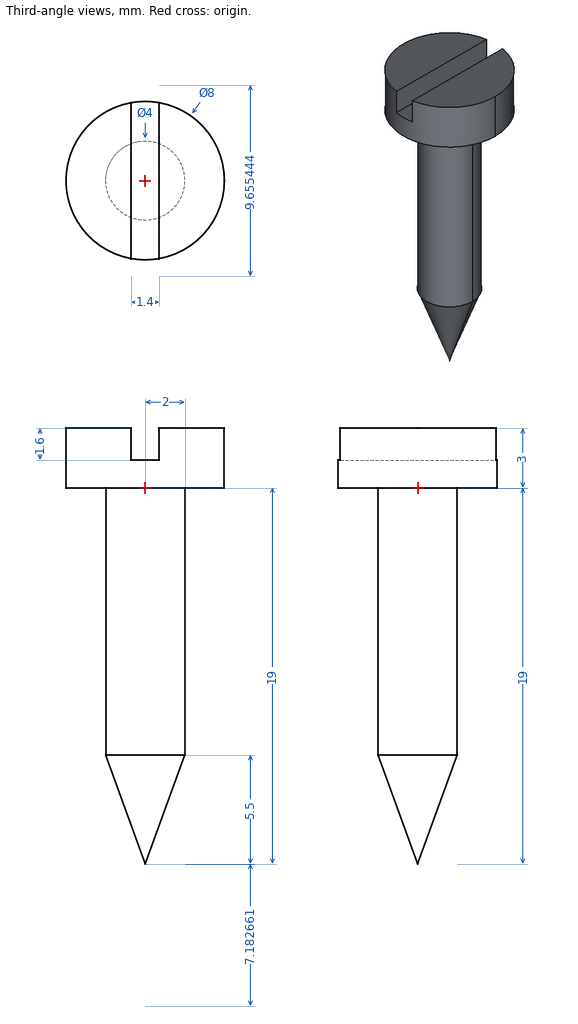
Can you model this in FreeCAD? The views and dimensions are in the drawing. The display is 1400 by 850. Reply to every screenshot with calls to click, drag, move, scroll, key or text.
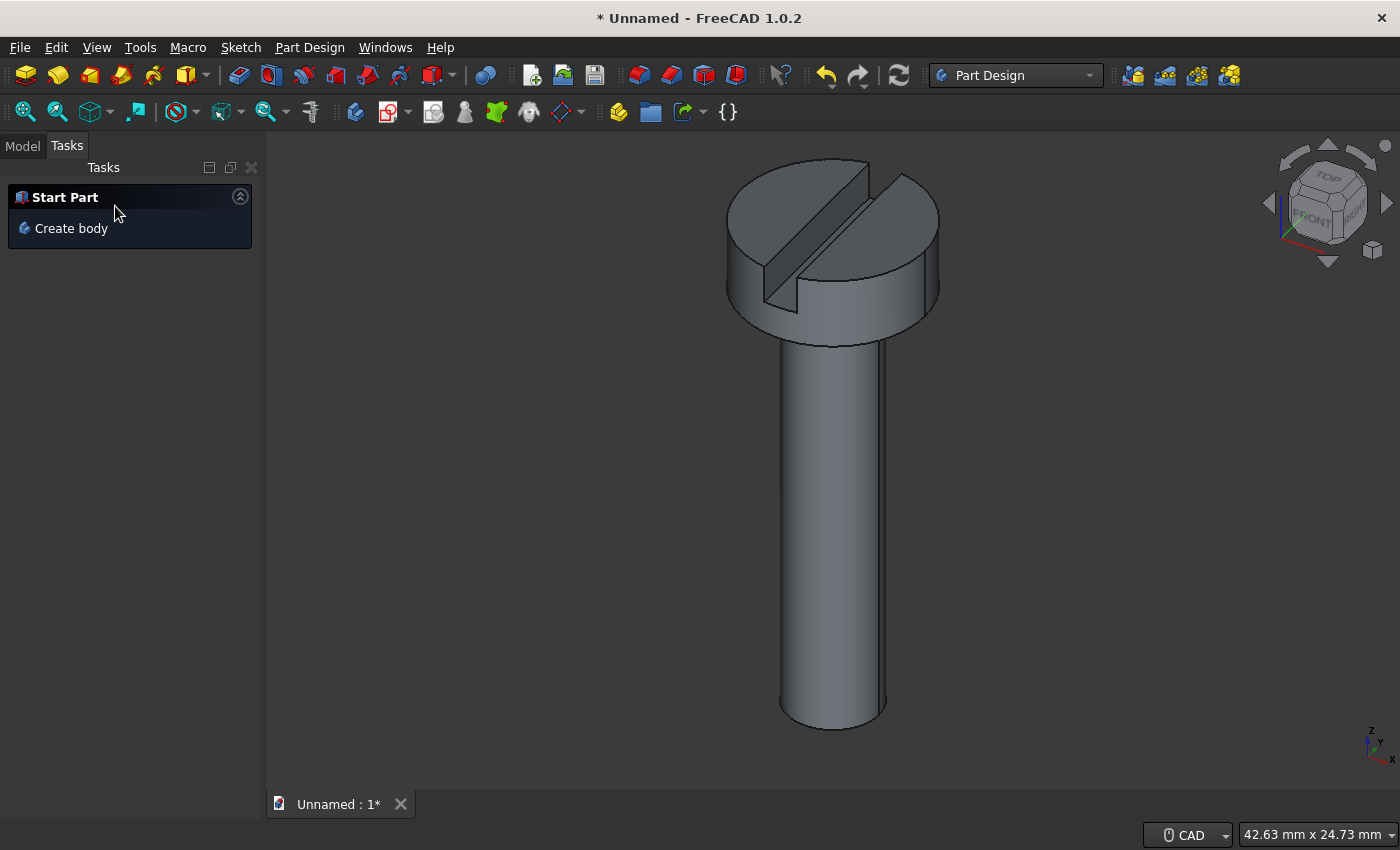
click(388, 112)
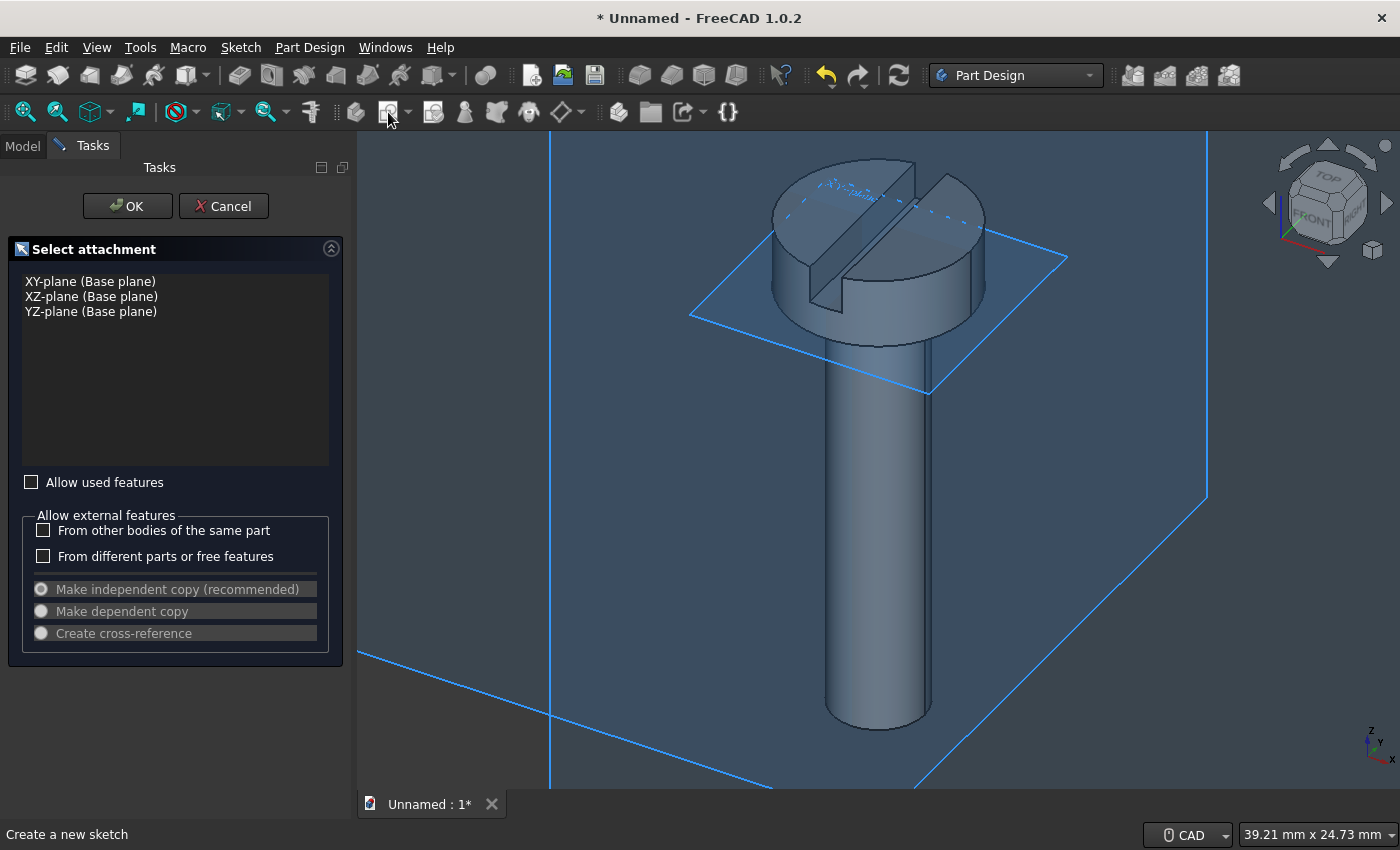
click(82, 296)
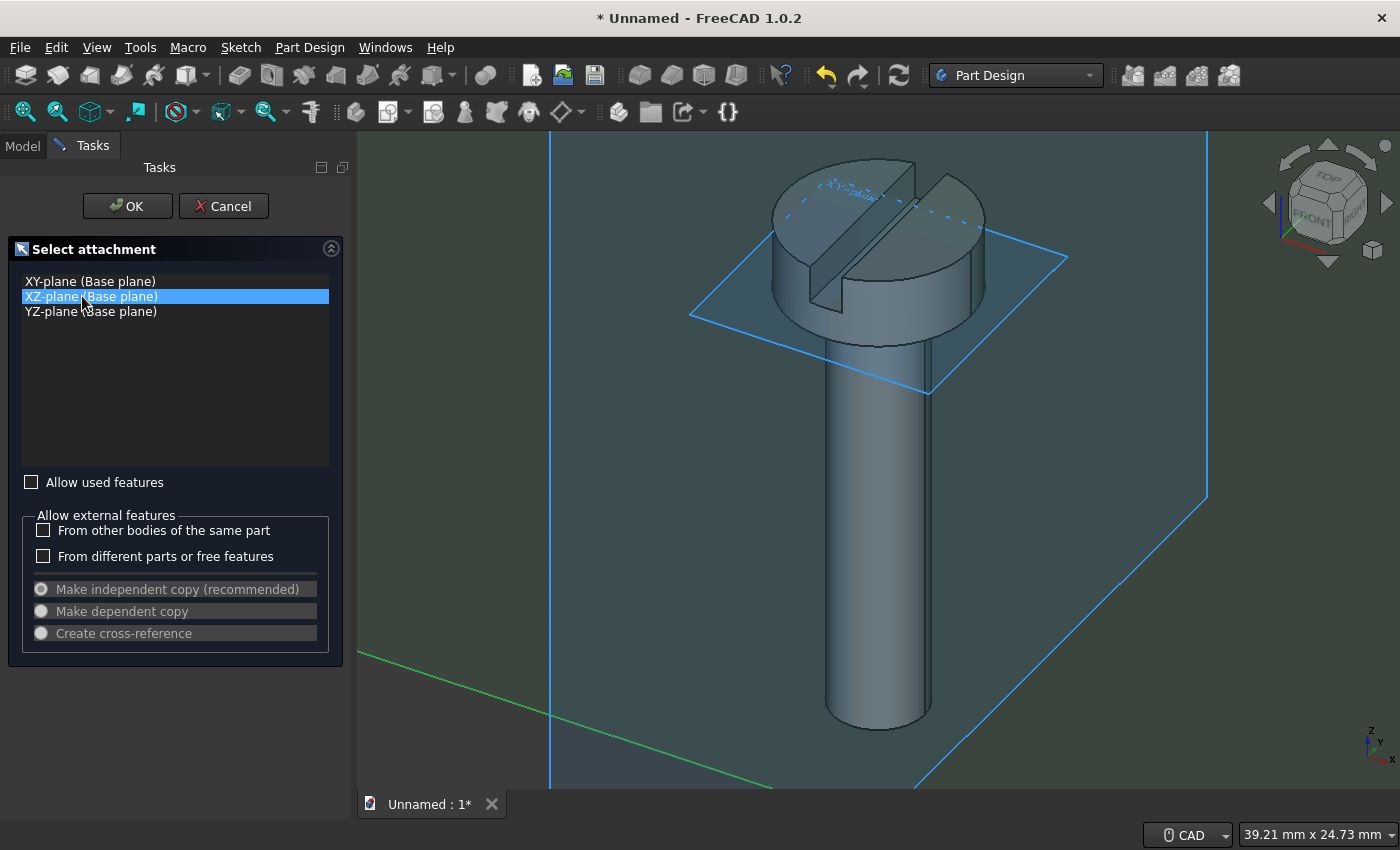
click(128, 206)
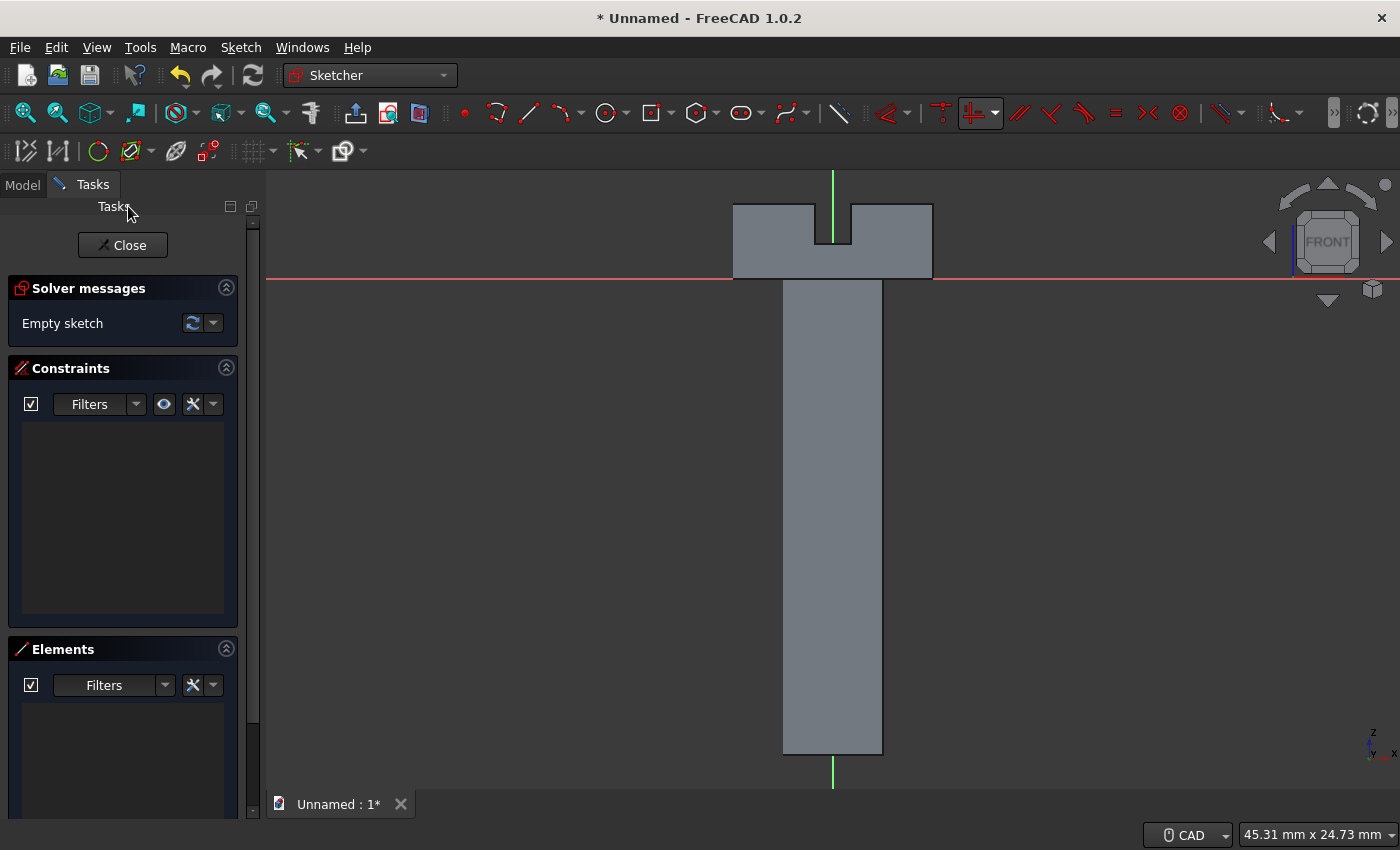
key(q)
key(s)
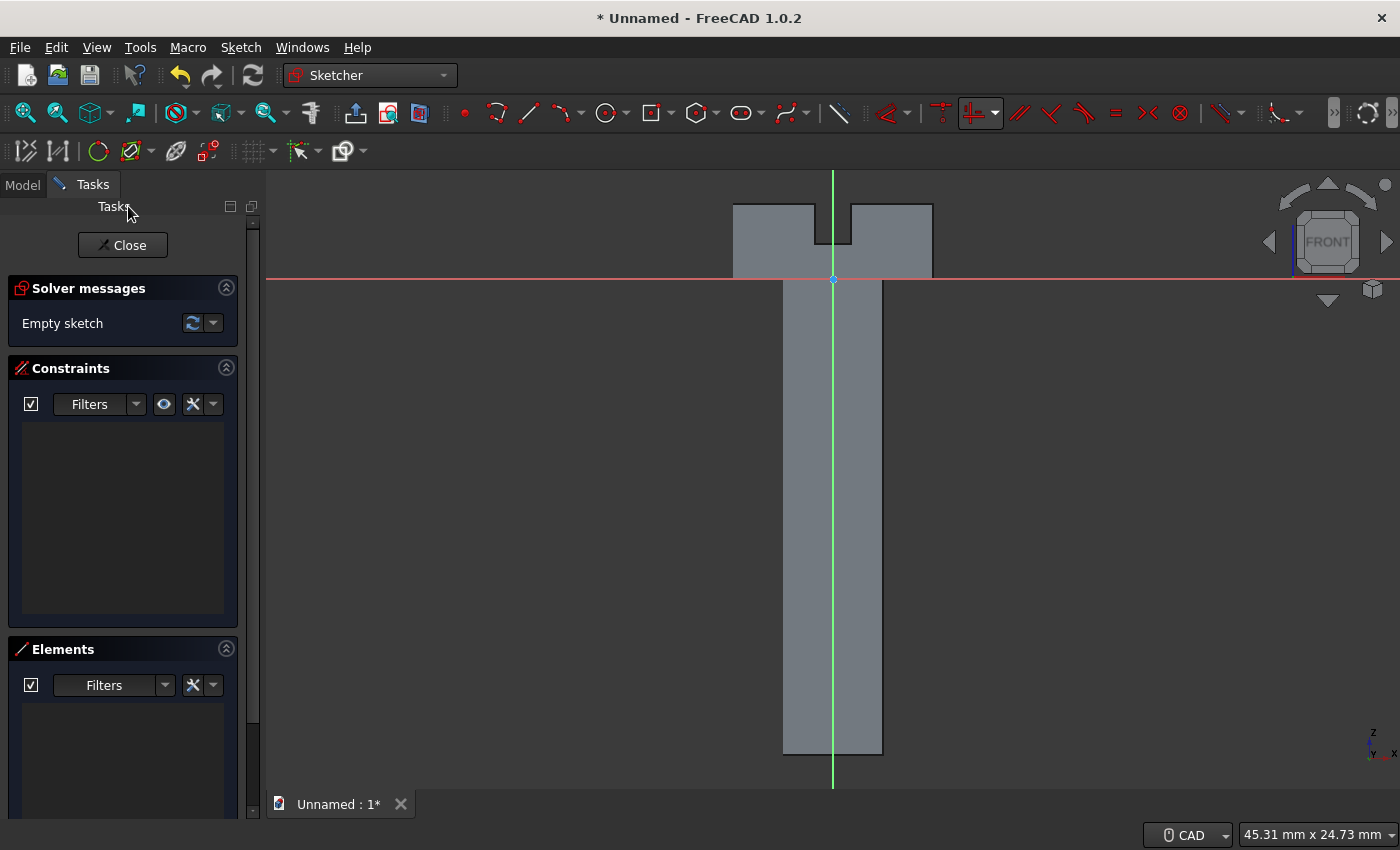
scroll(651, 325, down, 3)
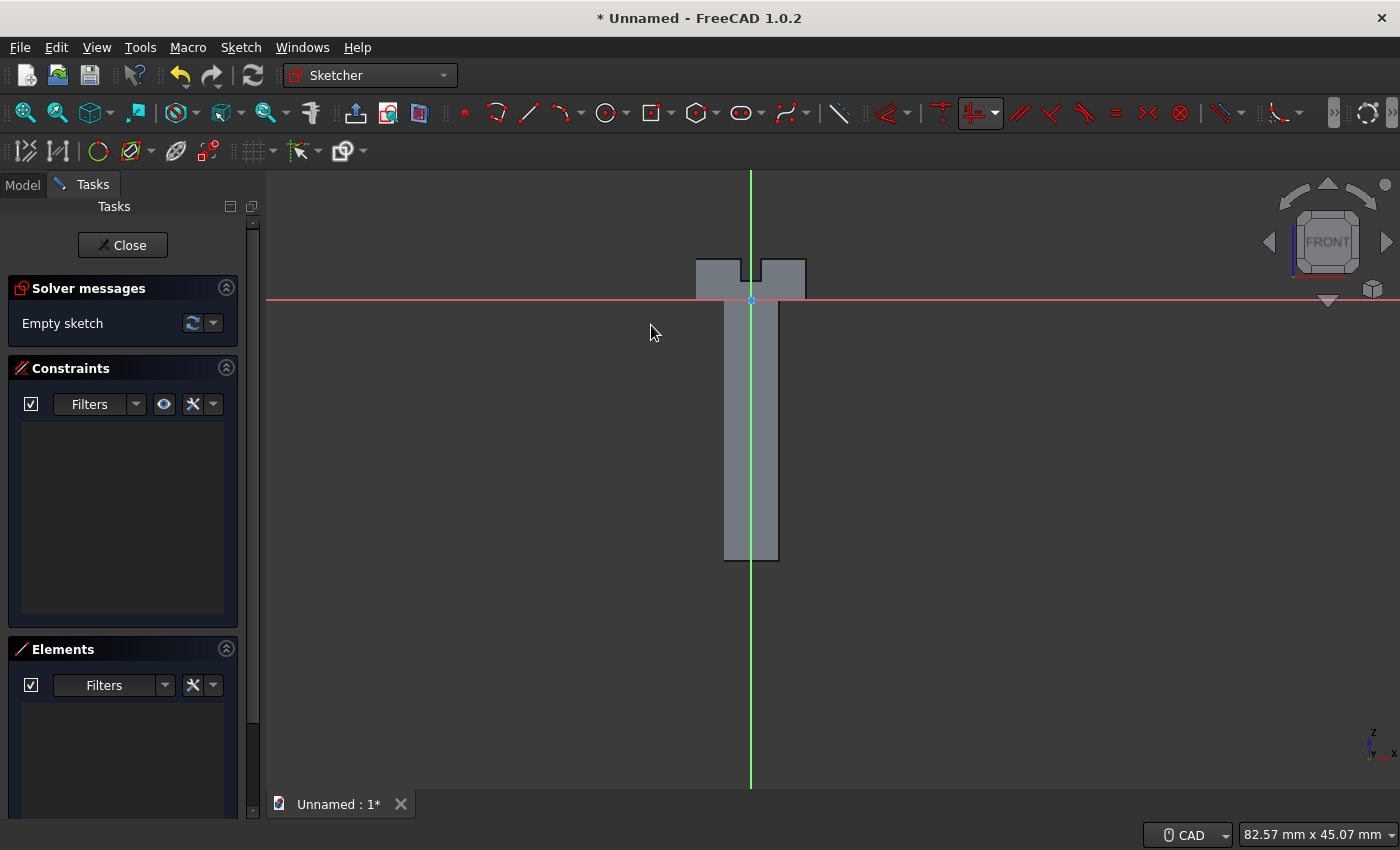
key(g)
key(m)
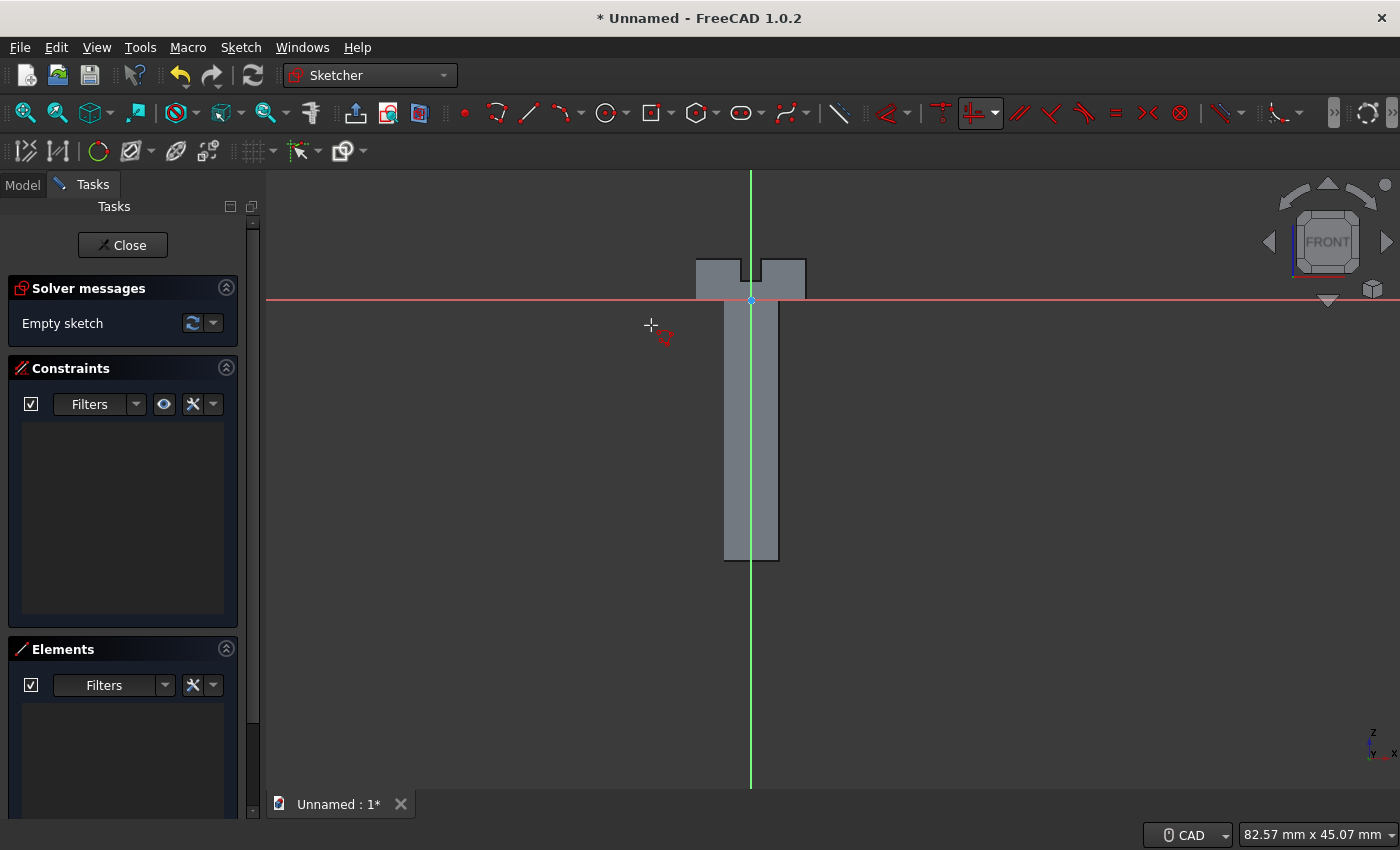
click(779, 485)
click(779, 561)
click(751, 660)
click(760, 561)
click(779, 486)
key(Escape)
key(Escape)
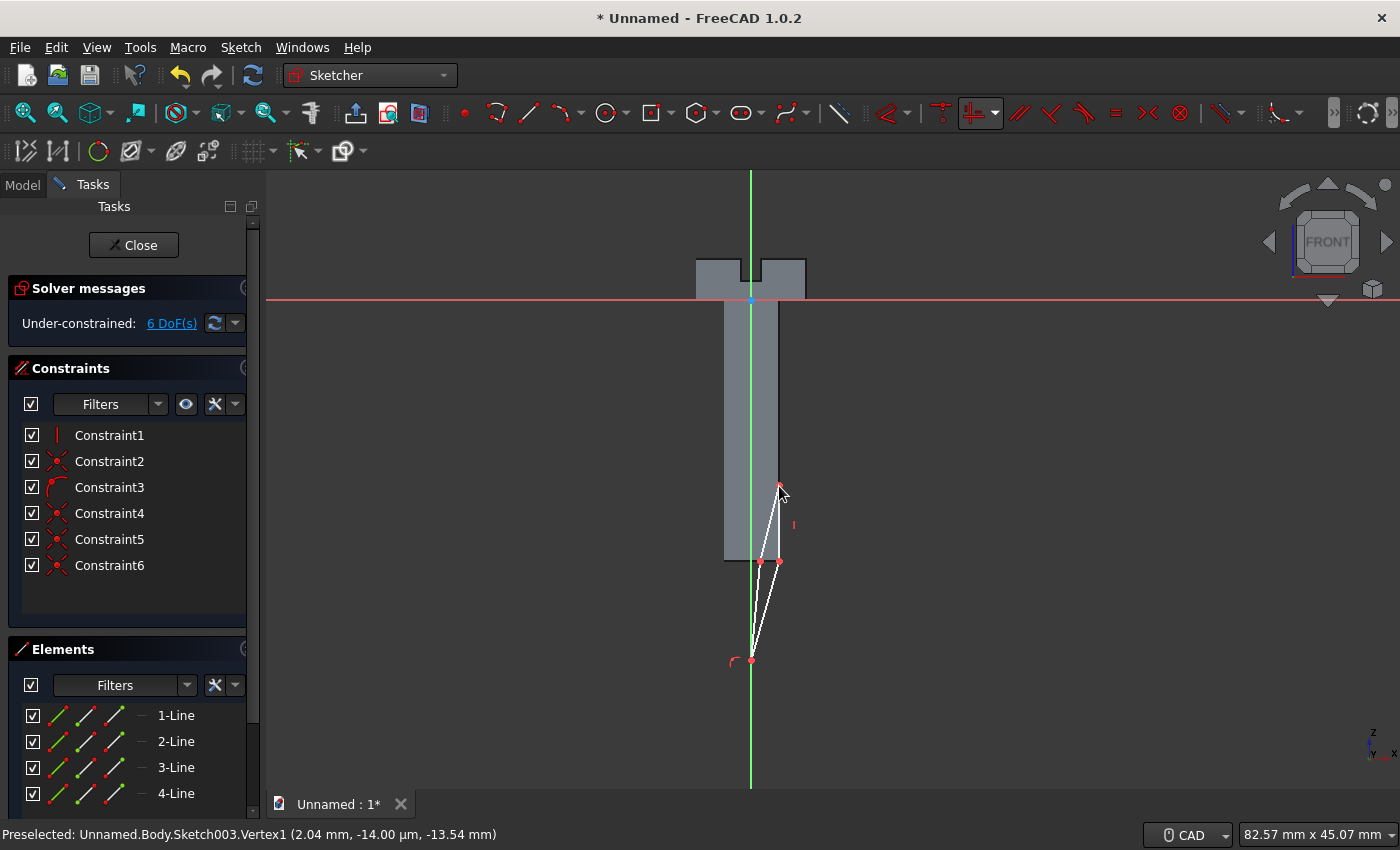
scroll(755, 621, up, 4)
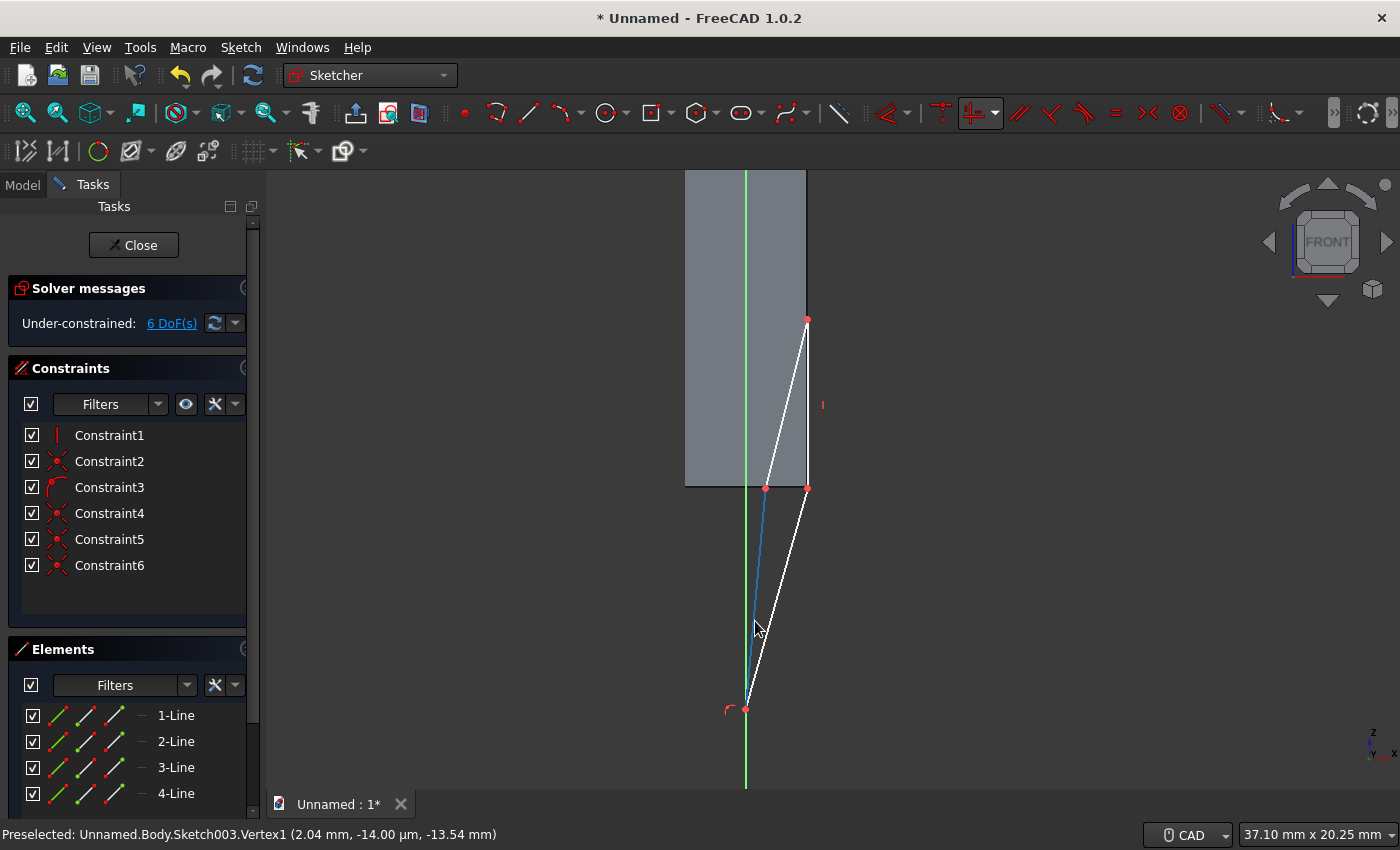
click(754, 621)